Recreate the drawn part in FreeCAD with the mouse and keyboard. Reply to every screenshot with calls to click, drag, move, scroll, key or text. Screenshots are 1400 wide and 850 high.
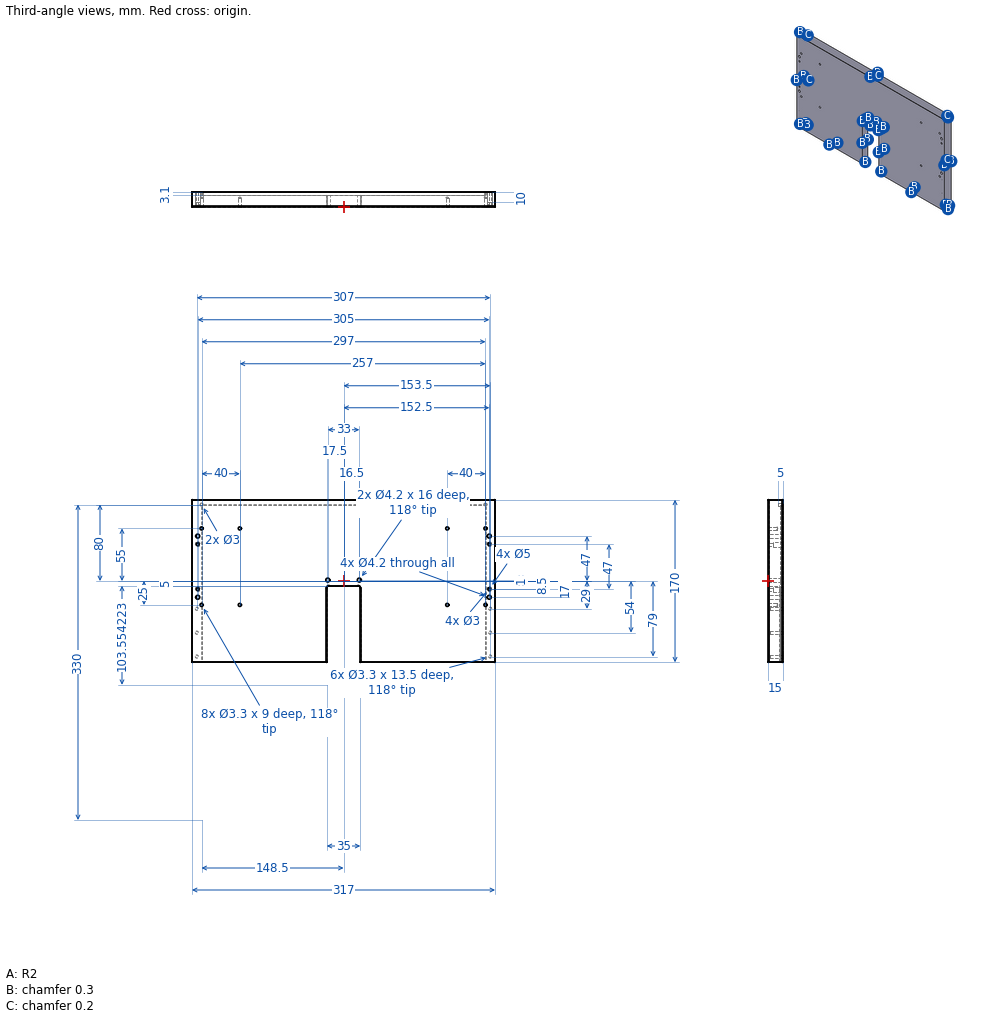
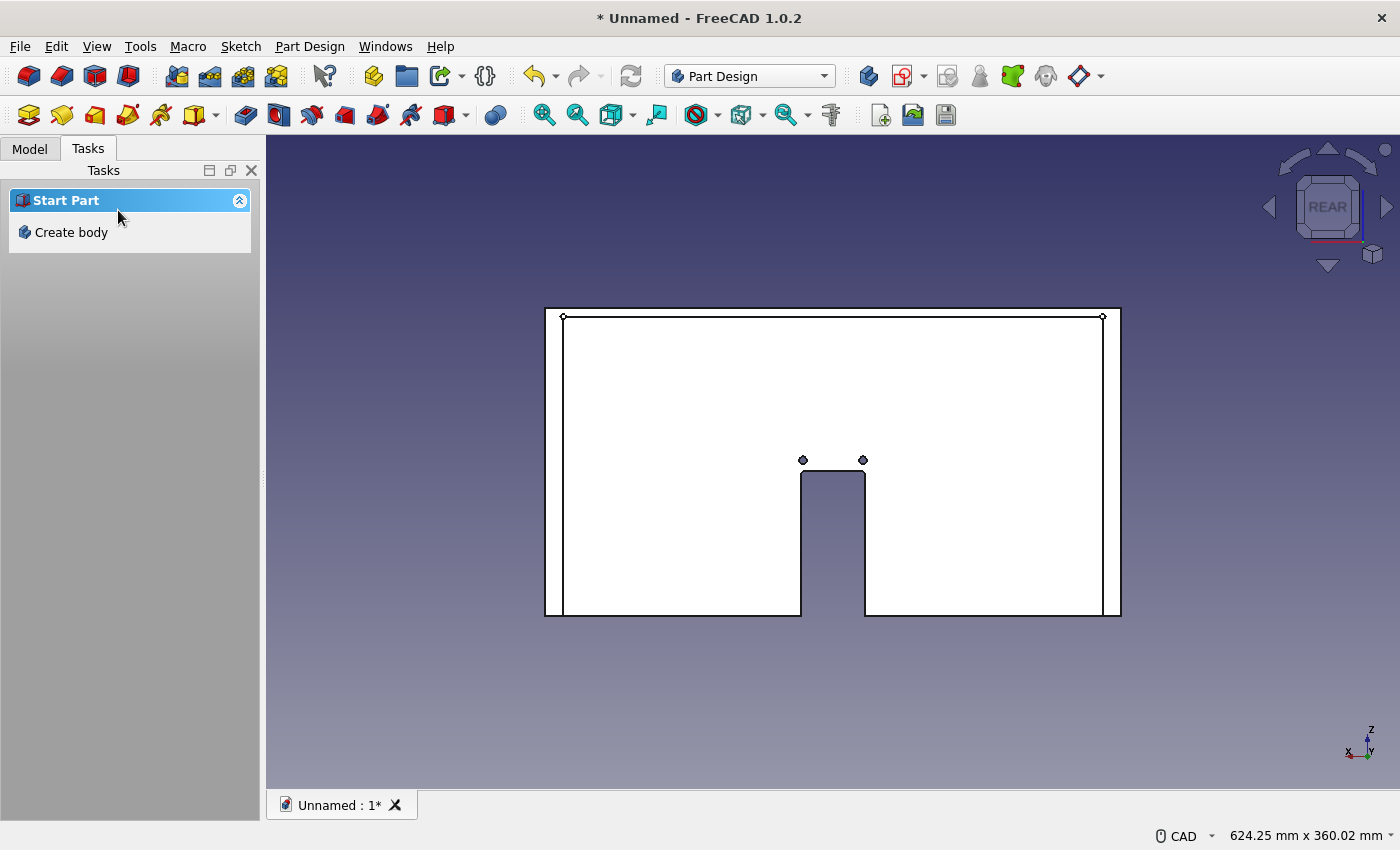
click(833, 470)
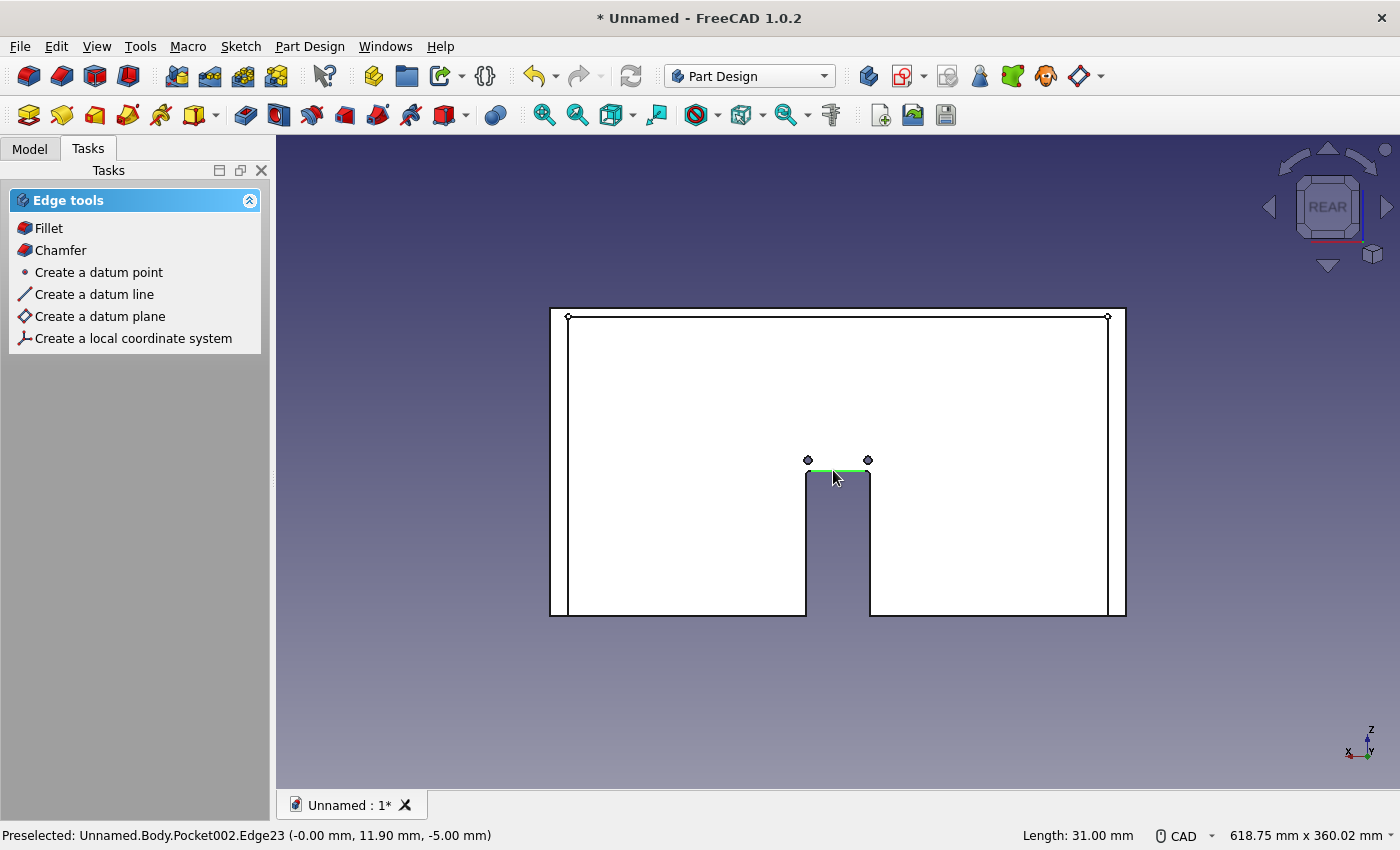
click(806, 545, ctrl)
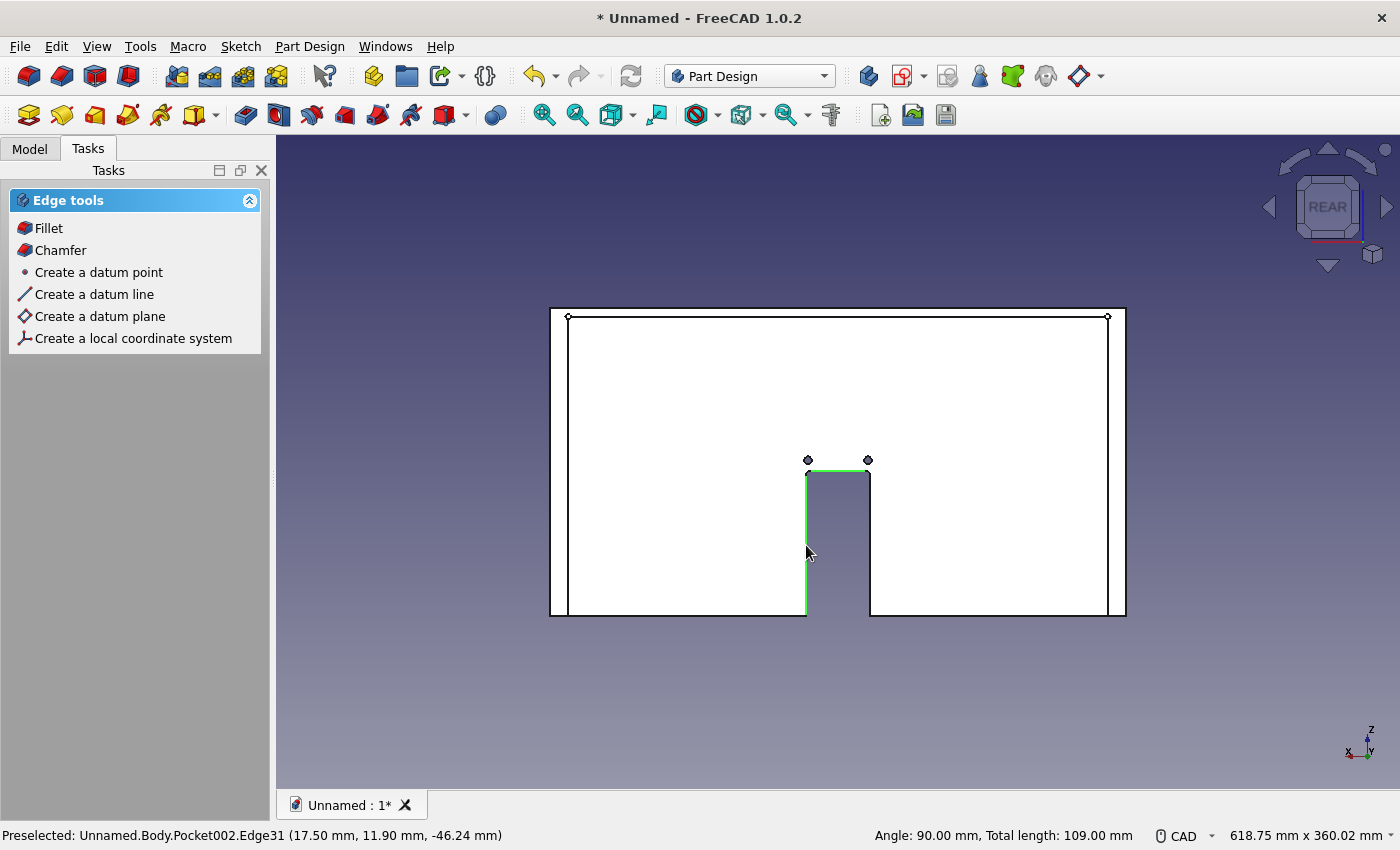
key(0)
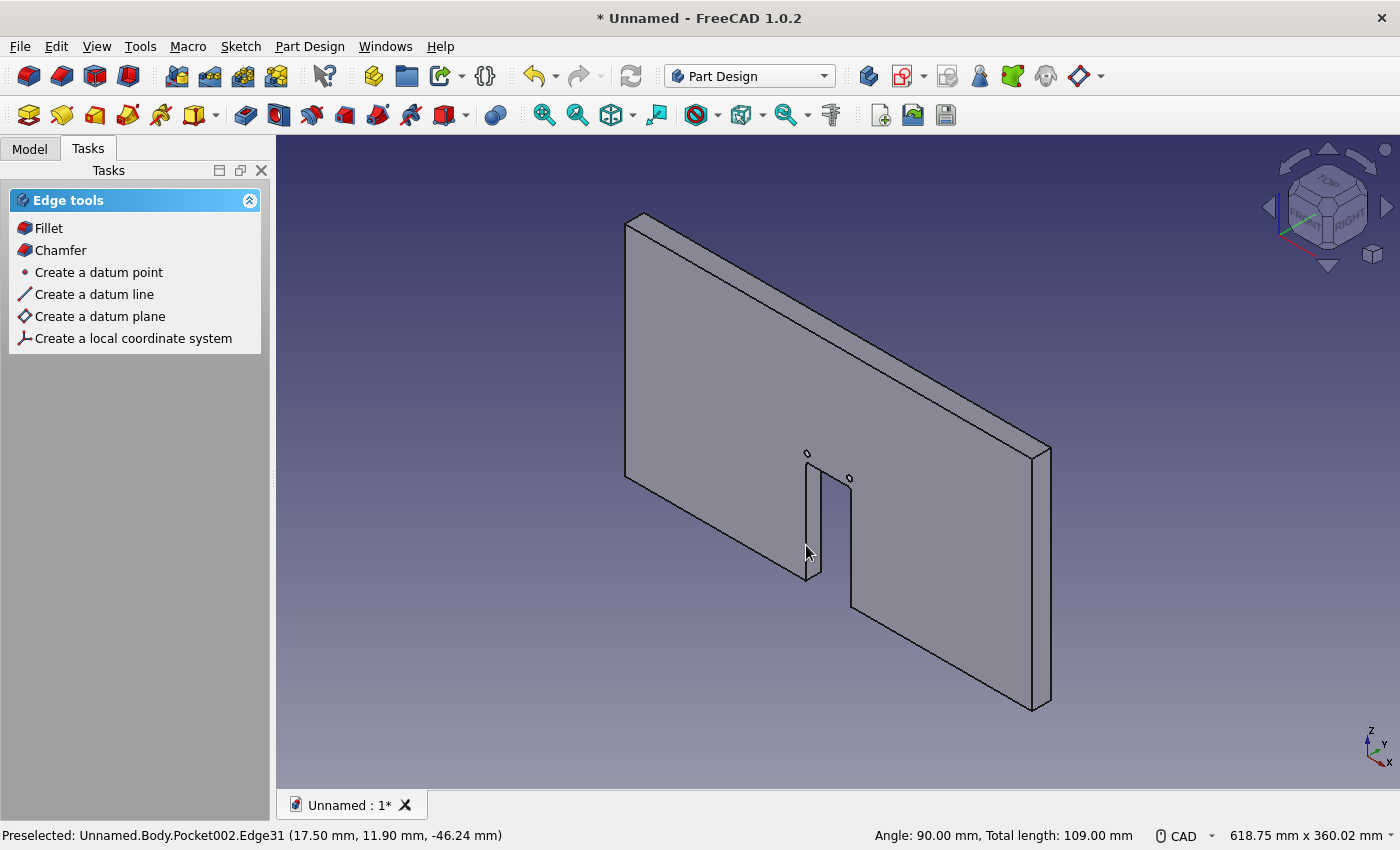
click(1013, 436, ctrl)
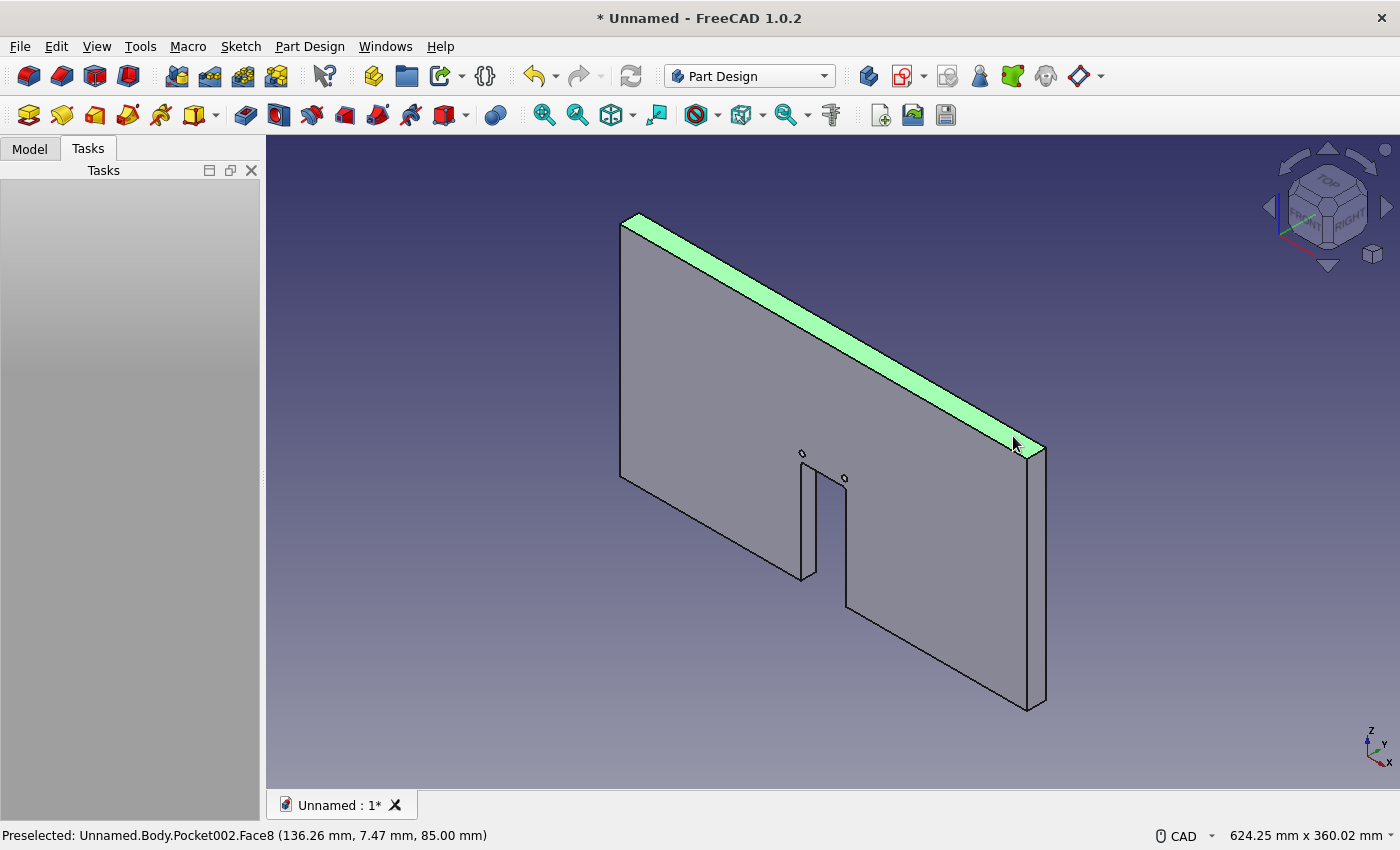
click(1037, 470, ctrl)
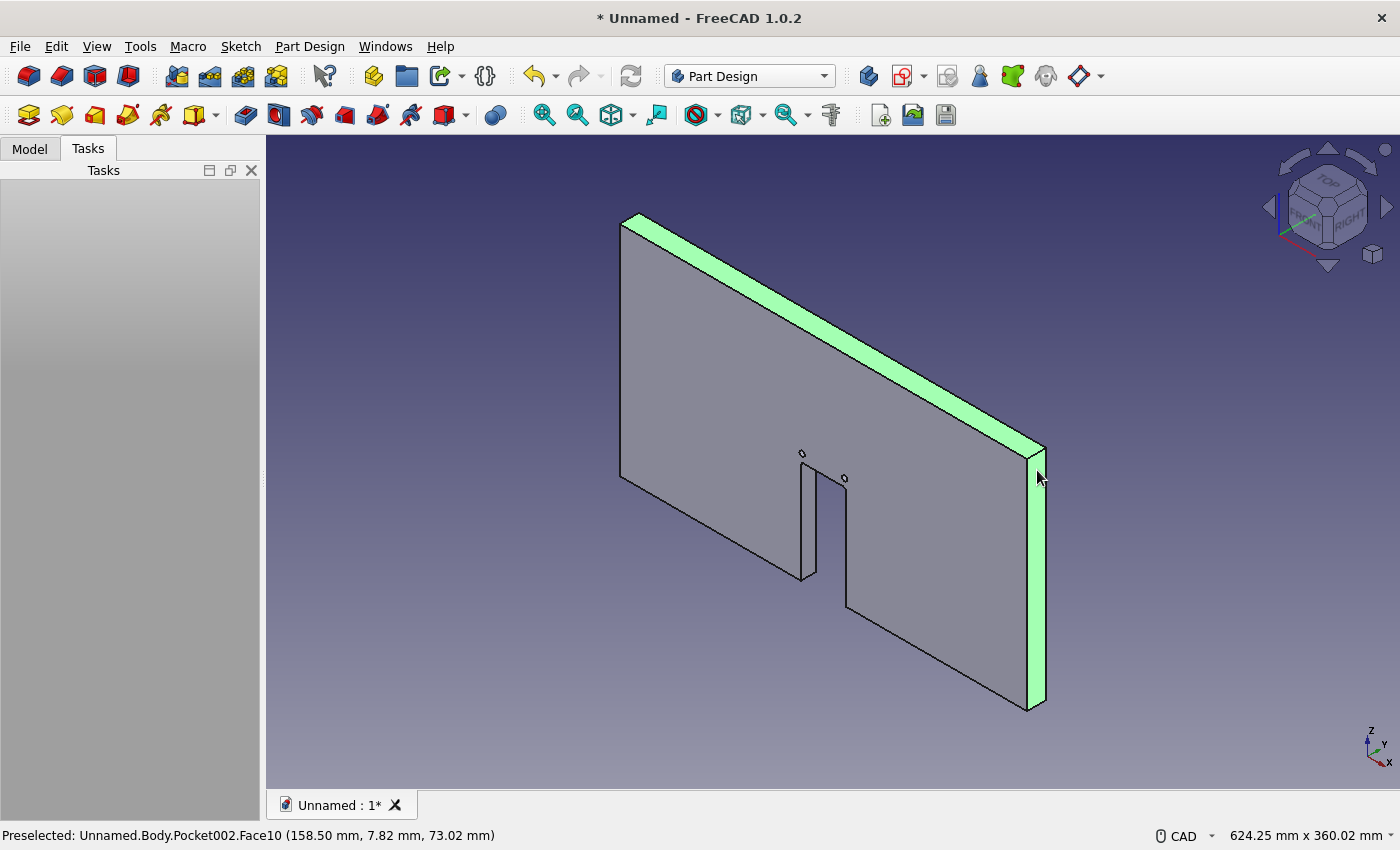
click(801, 522, ctrl)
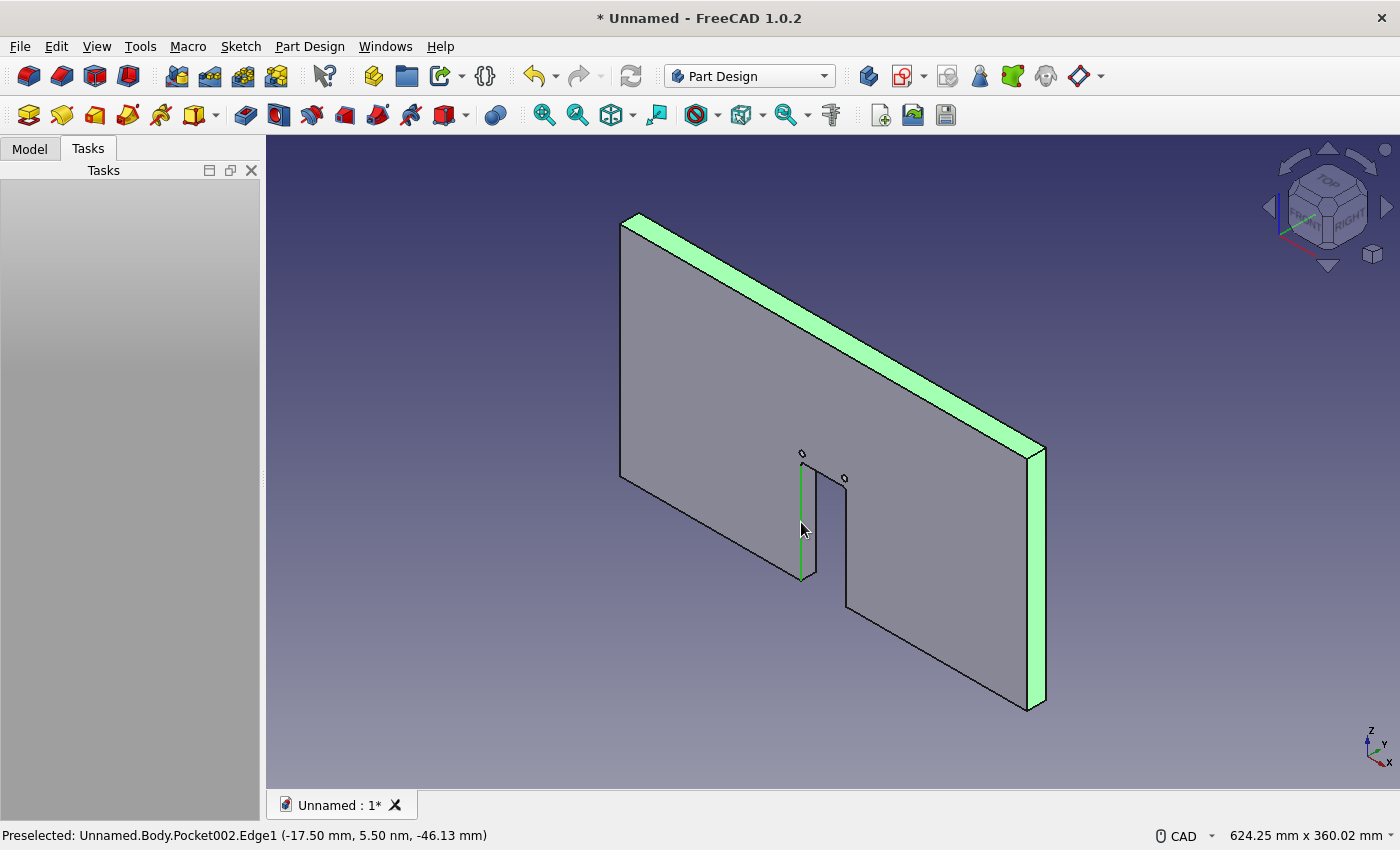
key(2)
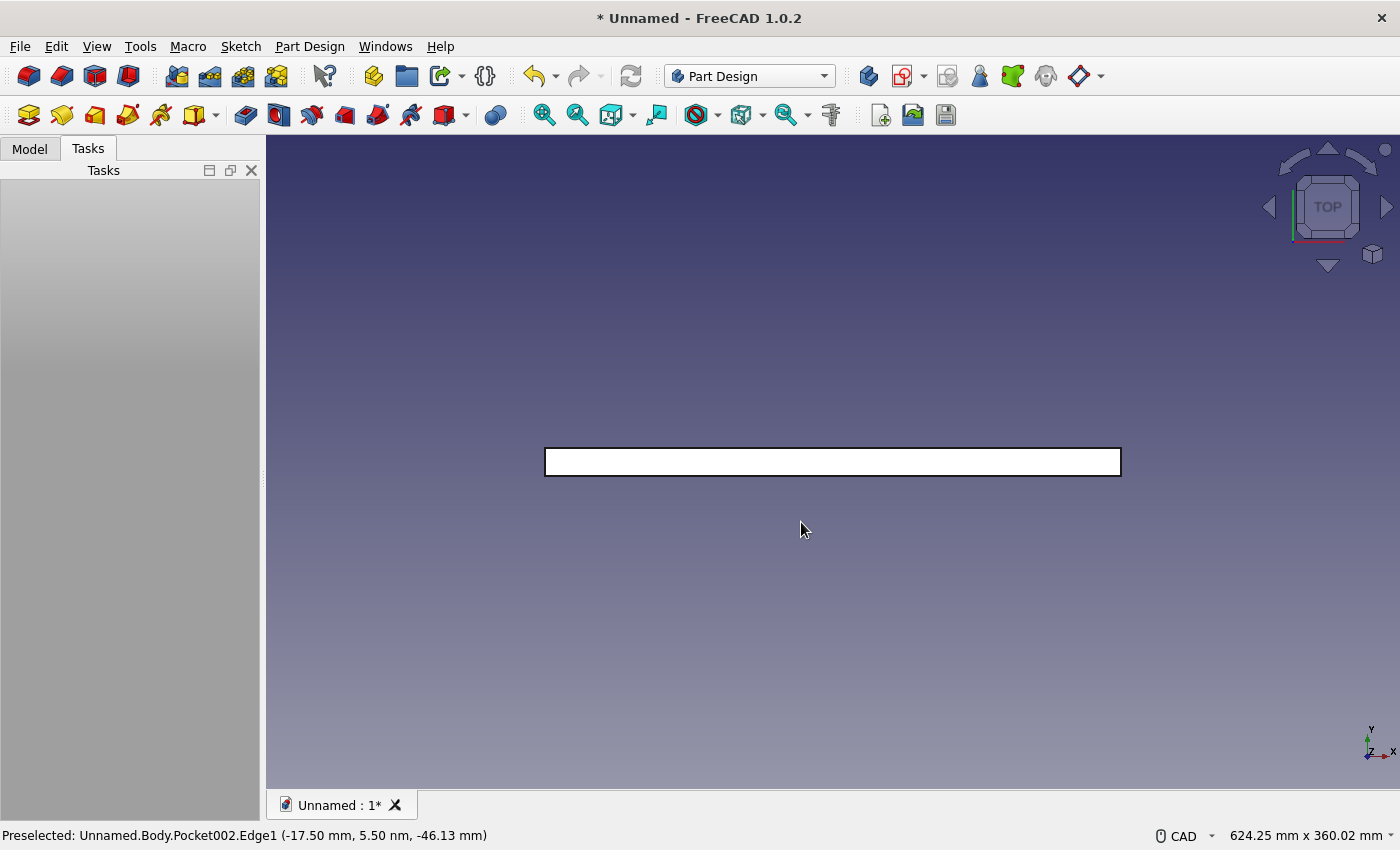
key(1)